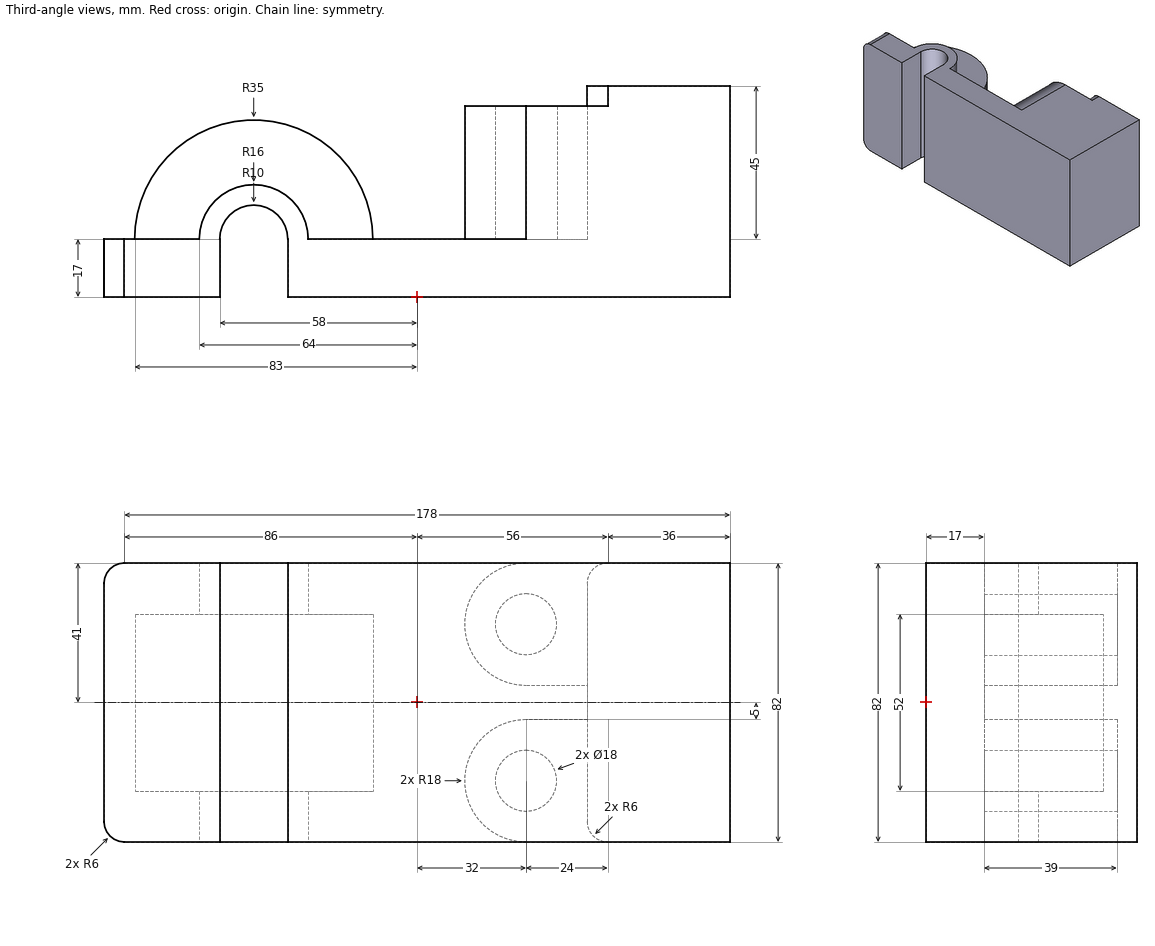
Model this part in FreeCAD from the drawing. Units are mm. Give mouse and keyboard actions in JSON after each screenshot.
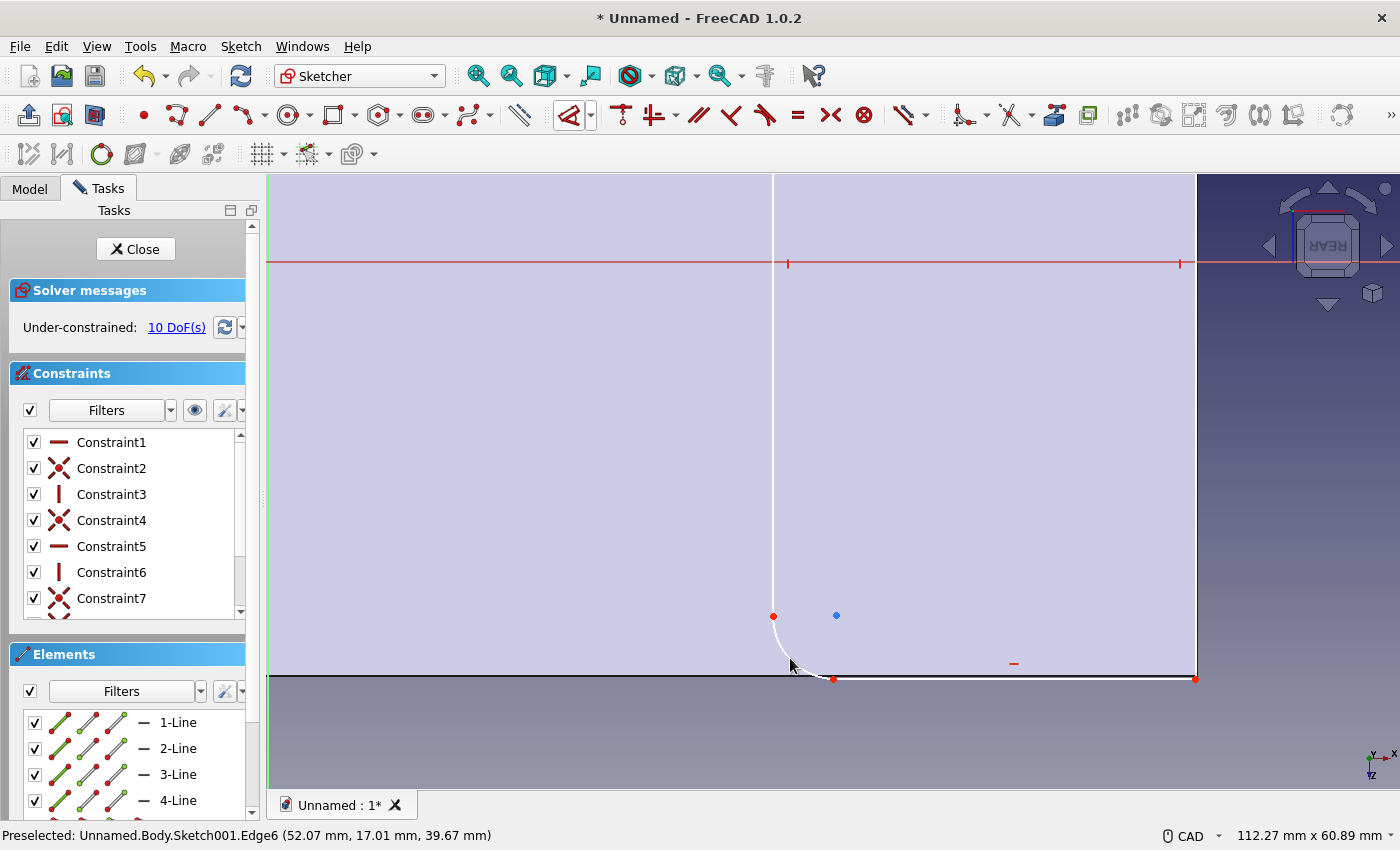
{"action": "left_click", "coordinate": [942, 679]}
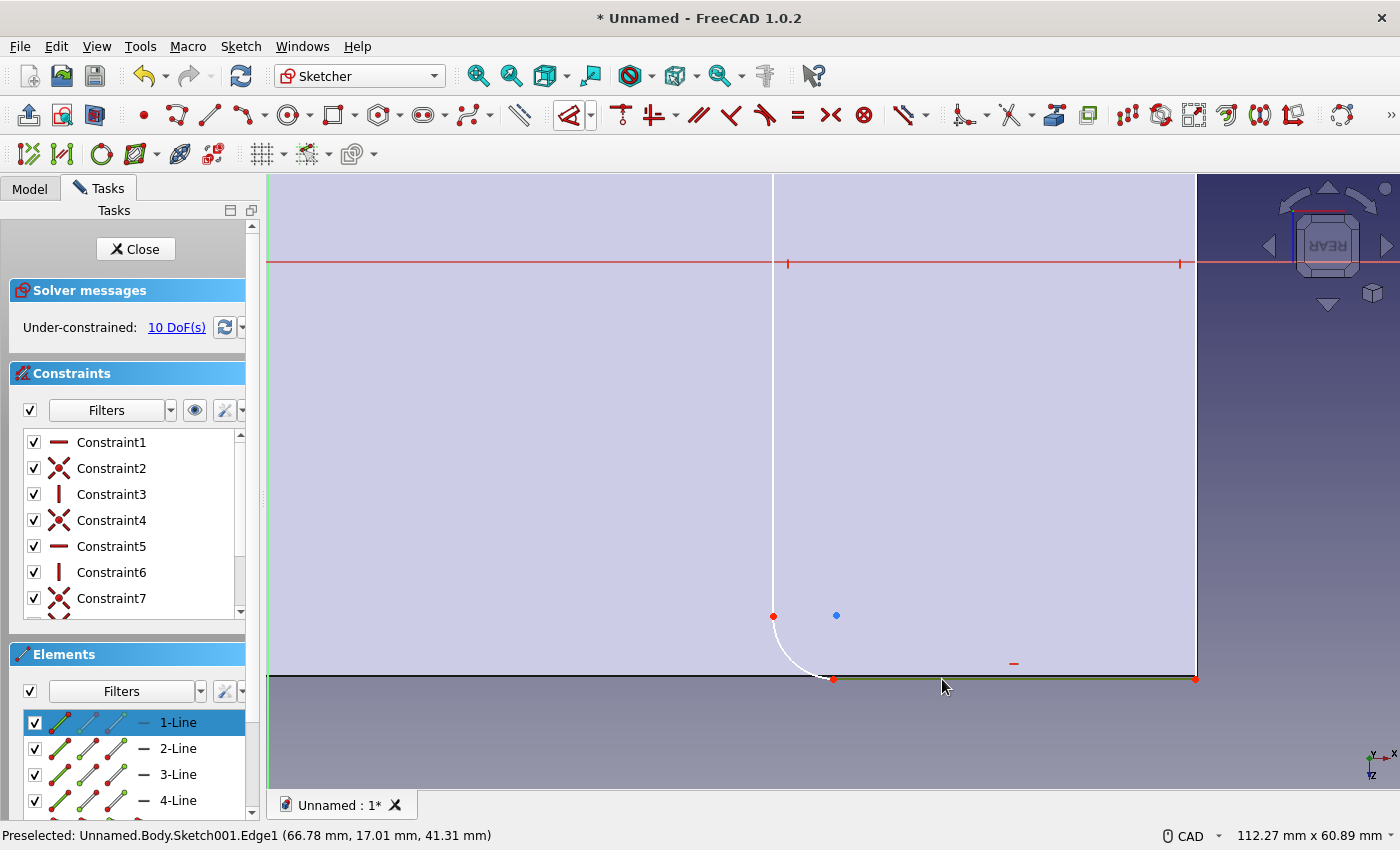
{"action": "left_click", "coordinate": [780, 644]}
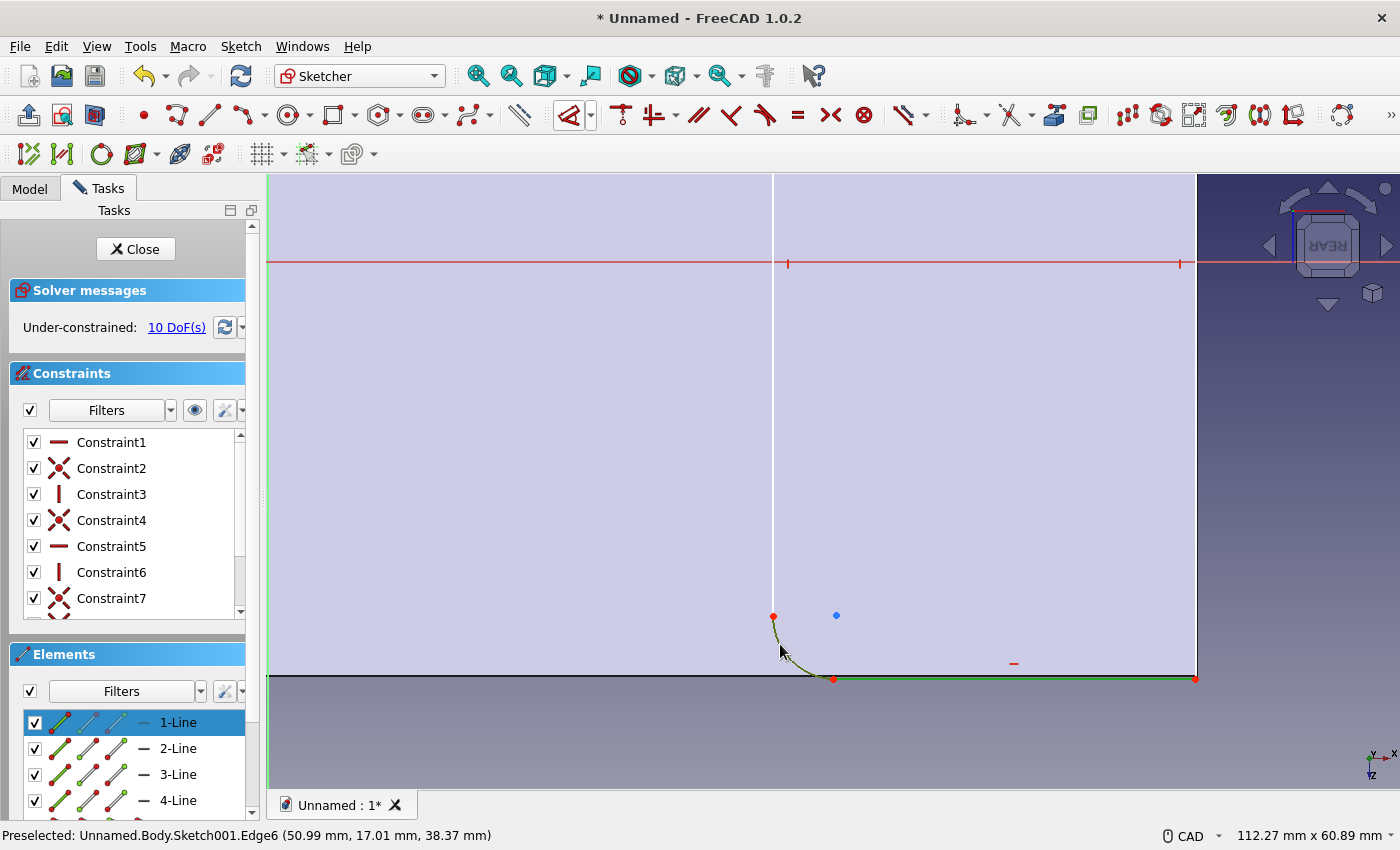
{"action": "left_click", "coordinate": [765, 116]}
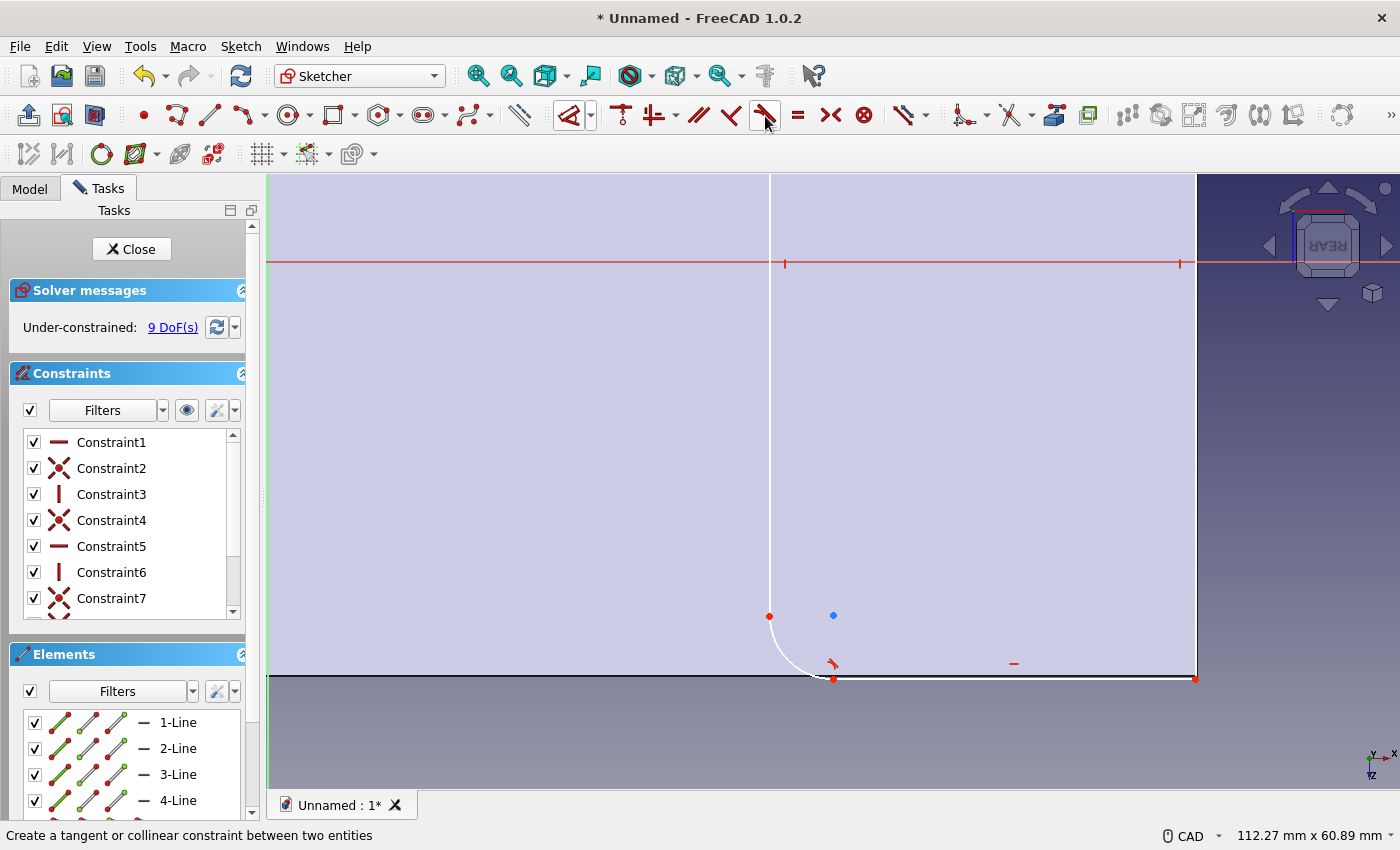
{"action": "scroll", "coordinate": [791, 661], "scroll_direction": "down", "scroll_amount": 4}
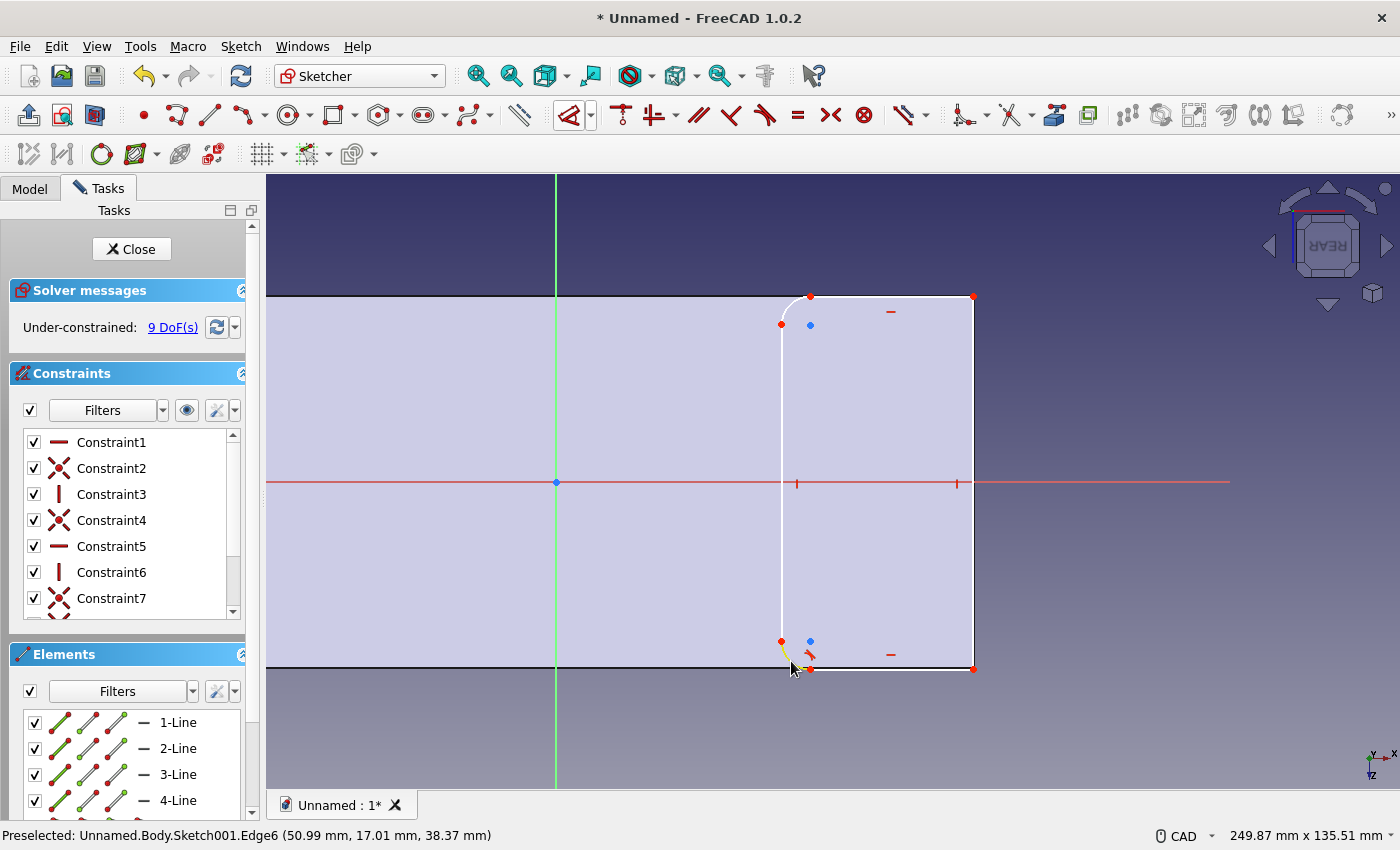
{"action": "left_click", "coordinate": [924, 297]}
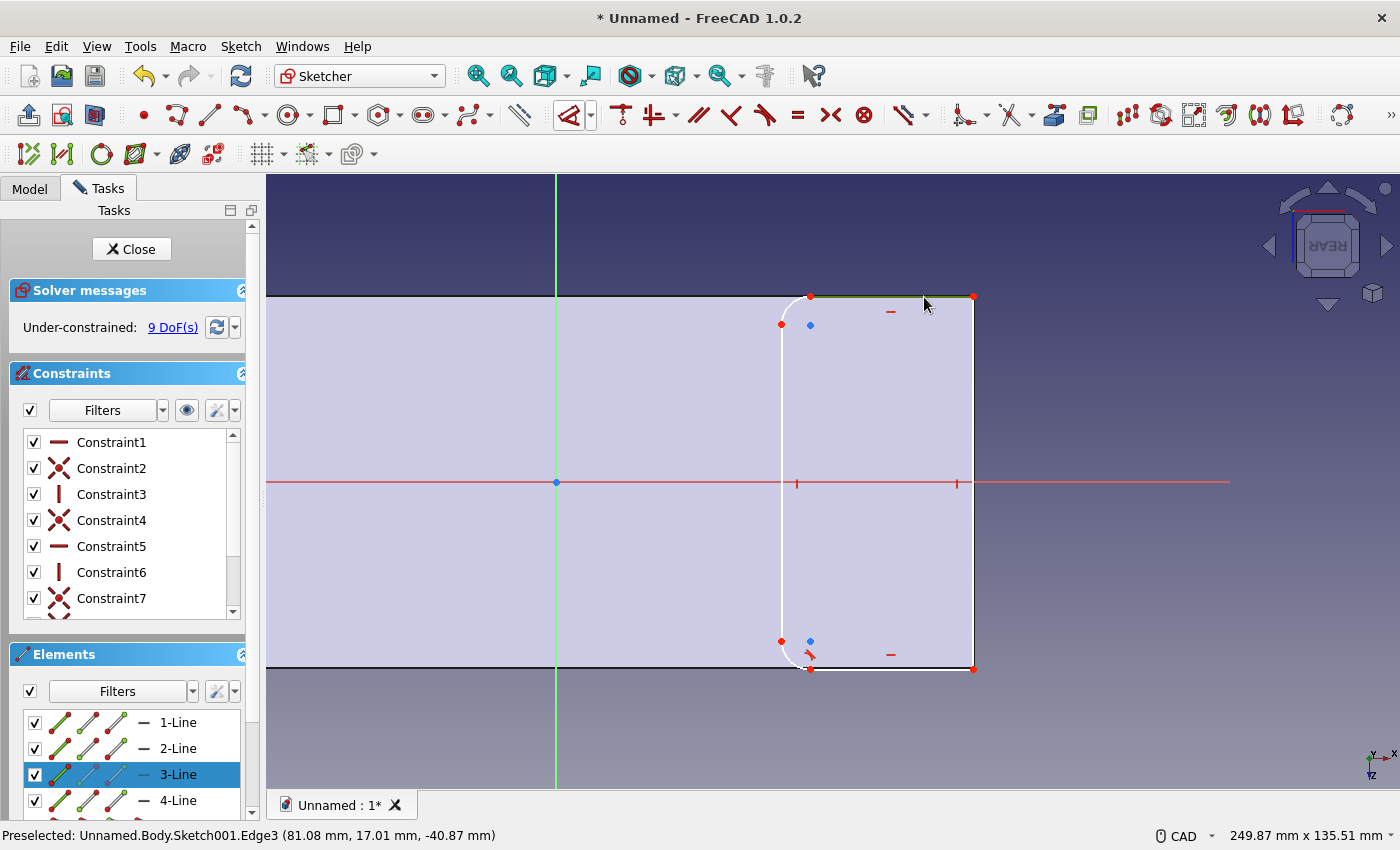
{"action": "left_click", "coordinate": [797, 300]}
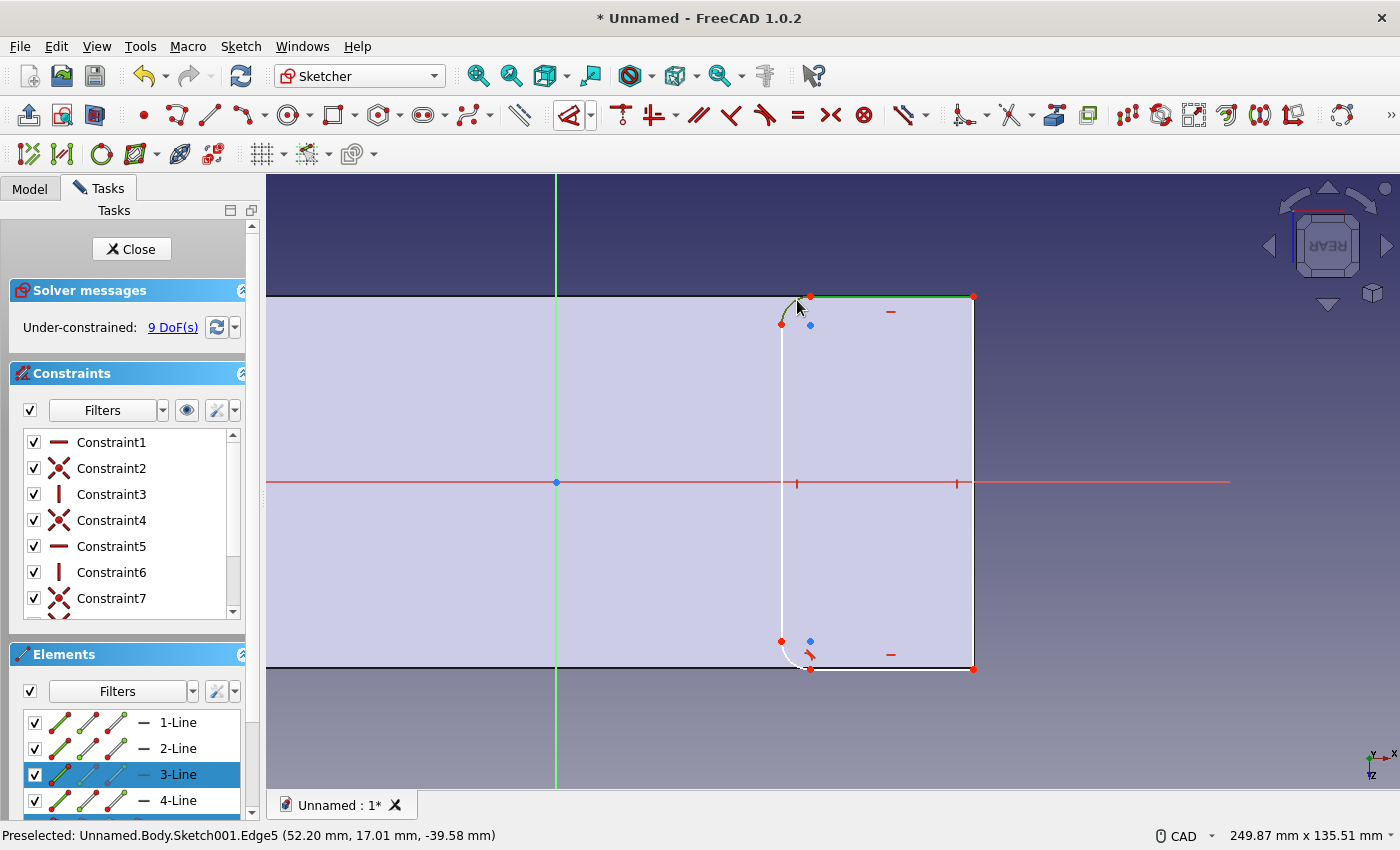
{"action": "left_click", "coordinate": [765, 116]}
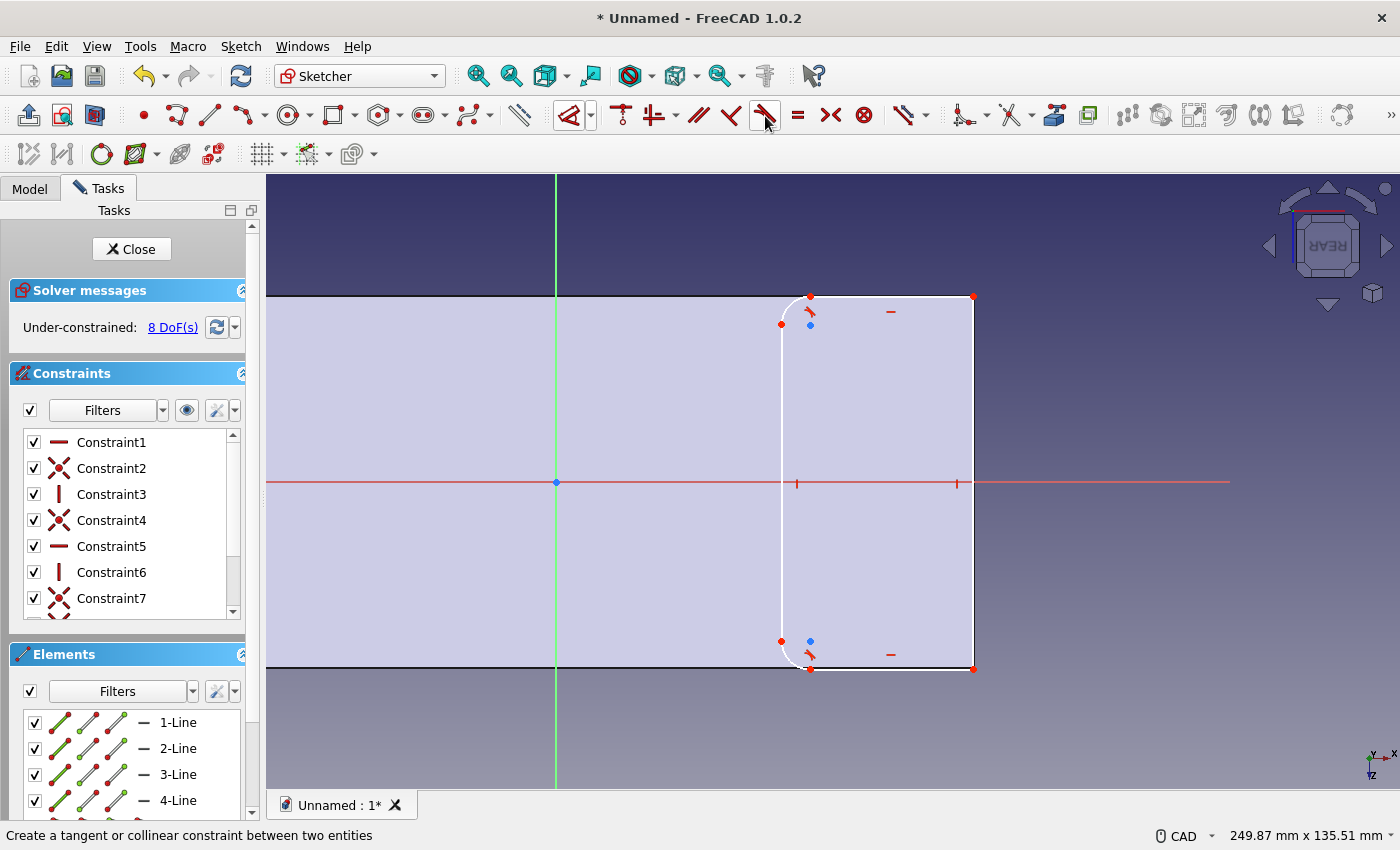
{"action": "left_click", "coordinate": [782, 420]}